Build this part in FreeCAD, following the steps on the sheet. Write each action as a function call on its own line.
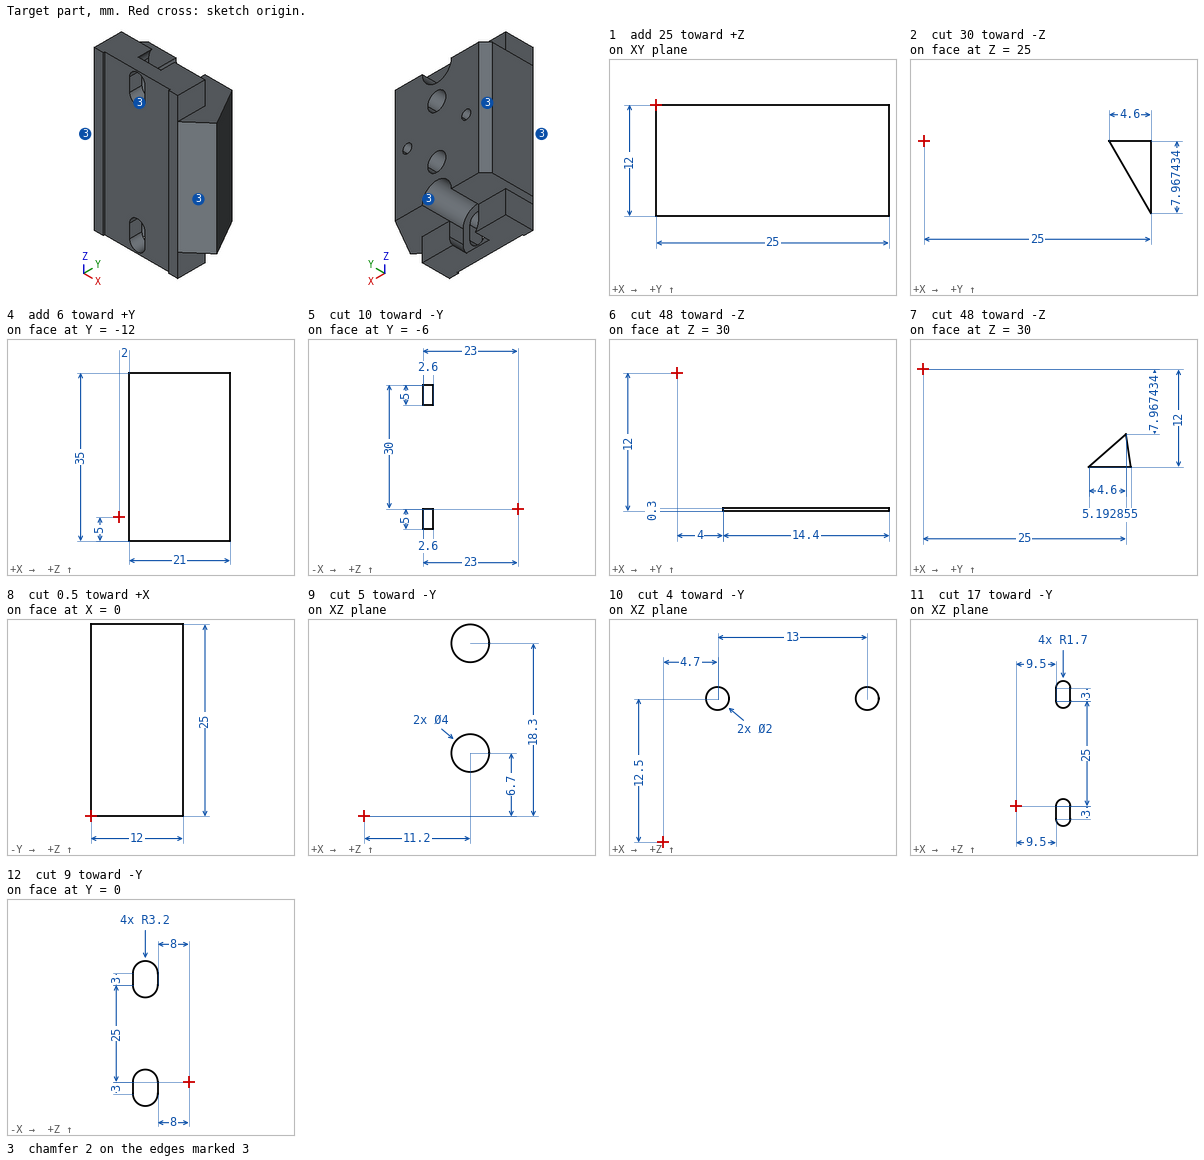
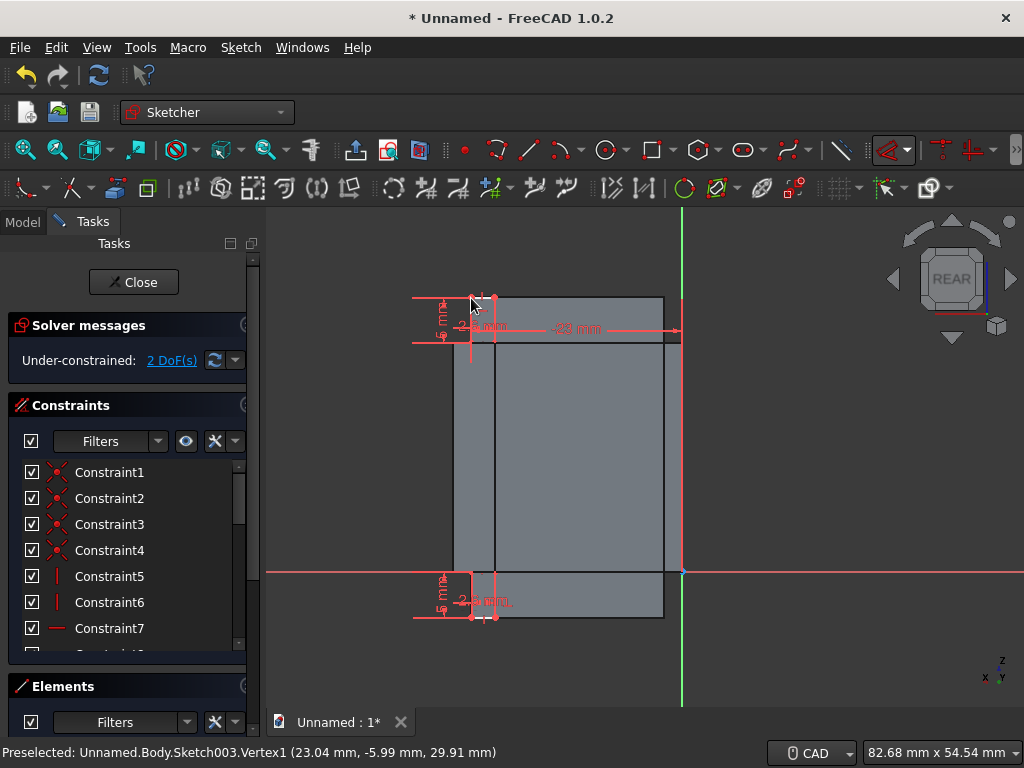
click(471, 298)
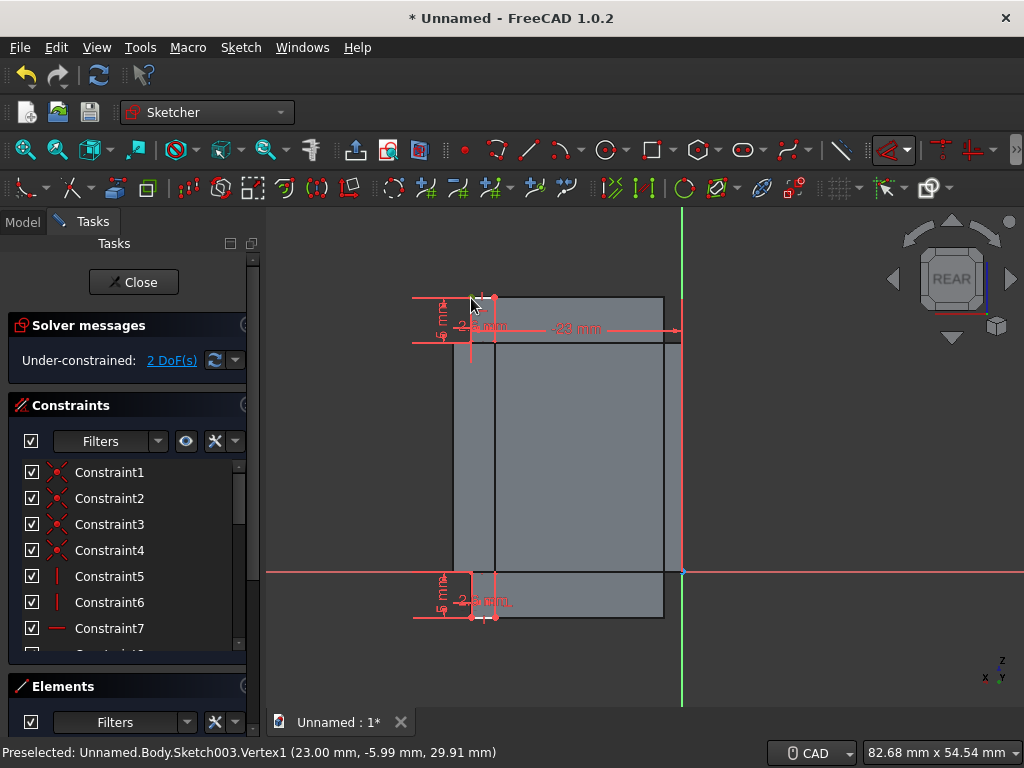
click(910, 150)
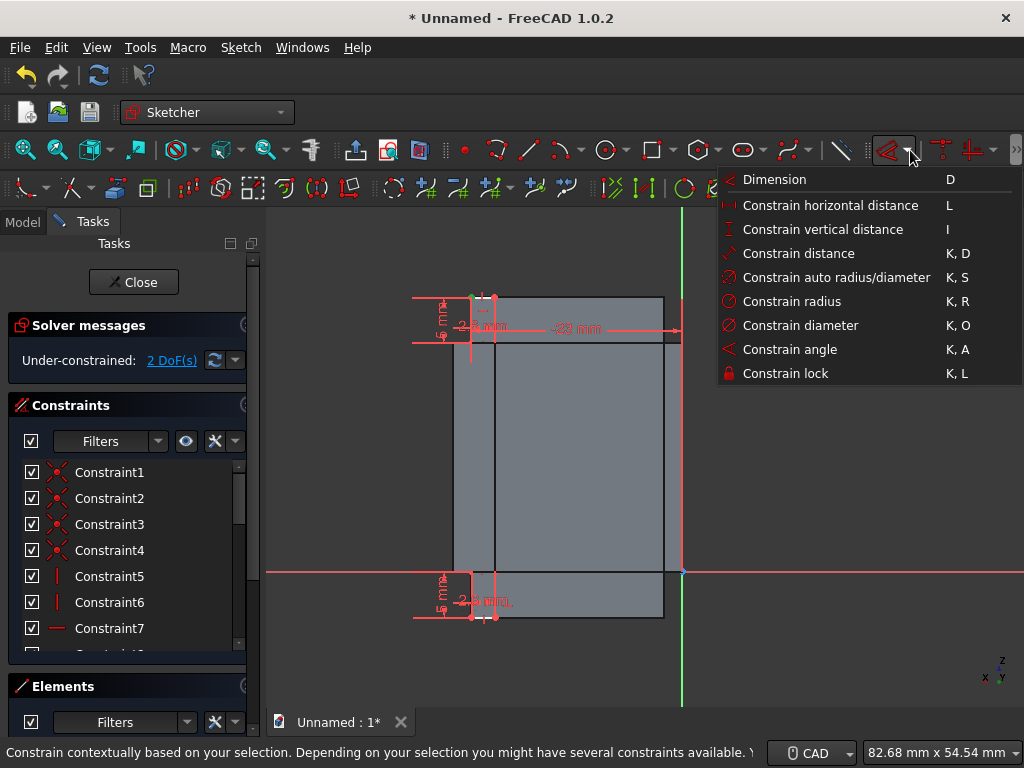
click(870, 229)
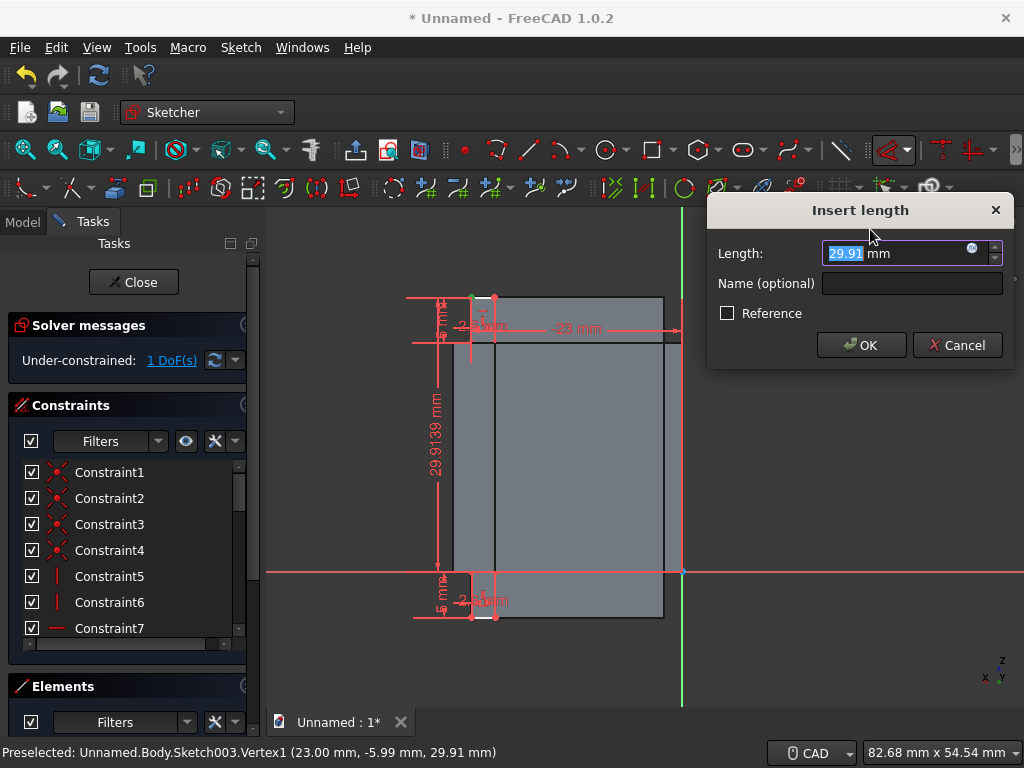
text(30)
key(Return)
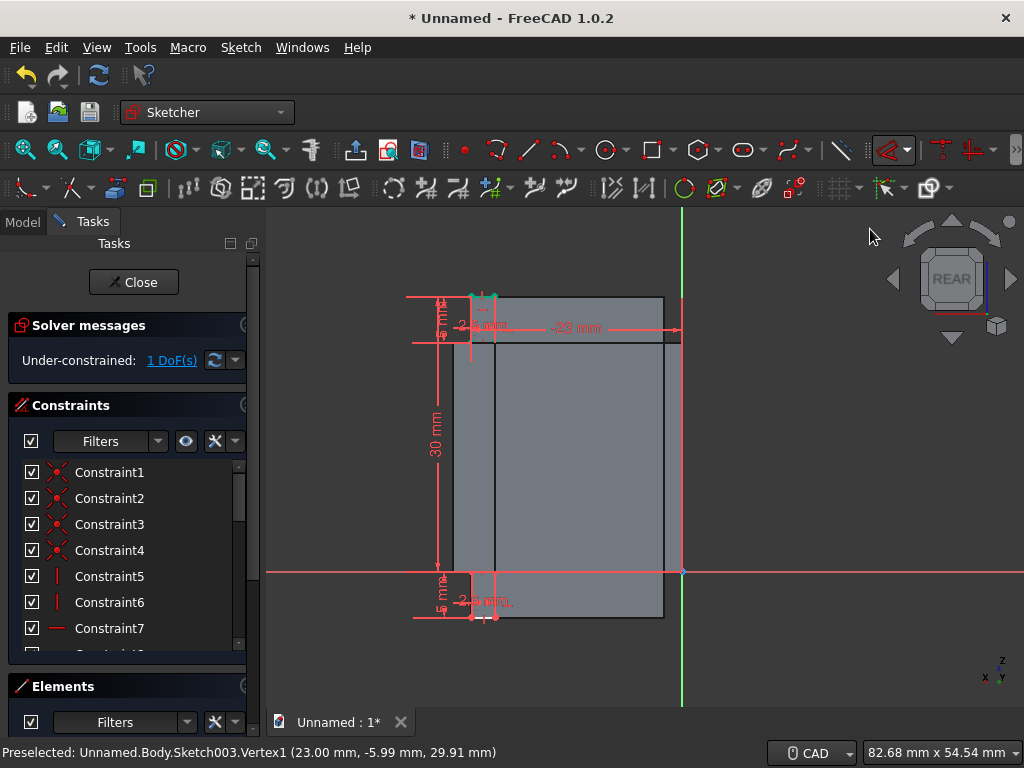
click(472, 572)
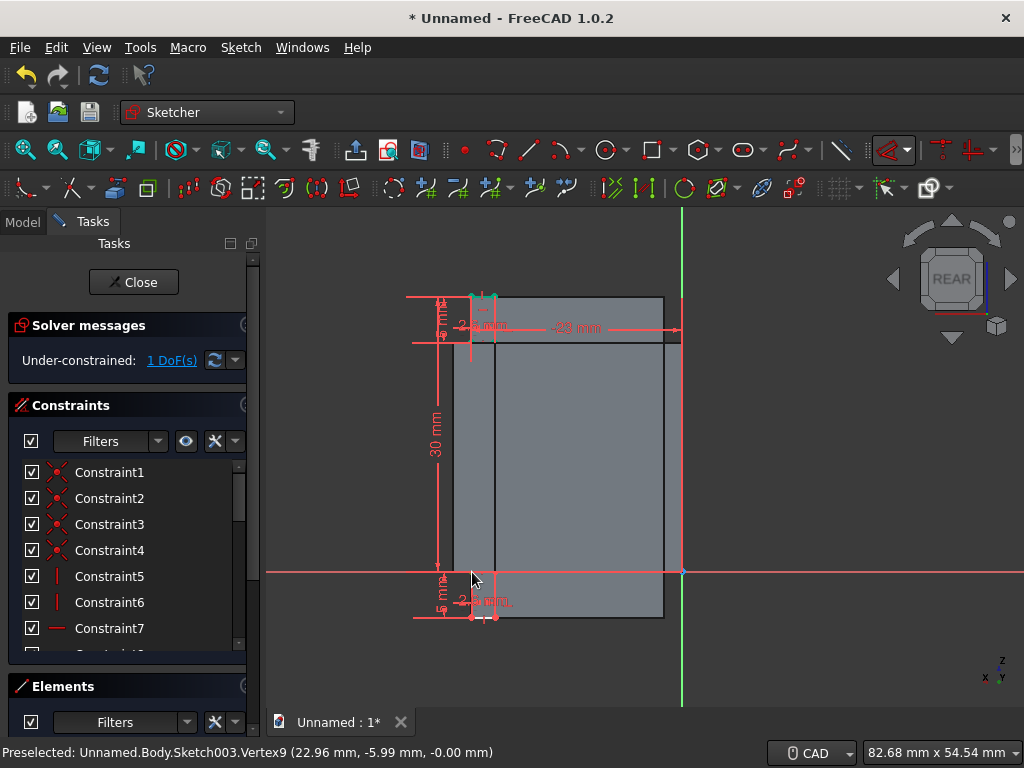
click(910, 150)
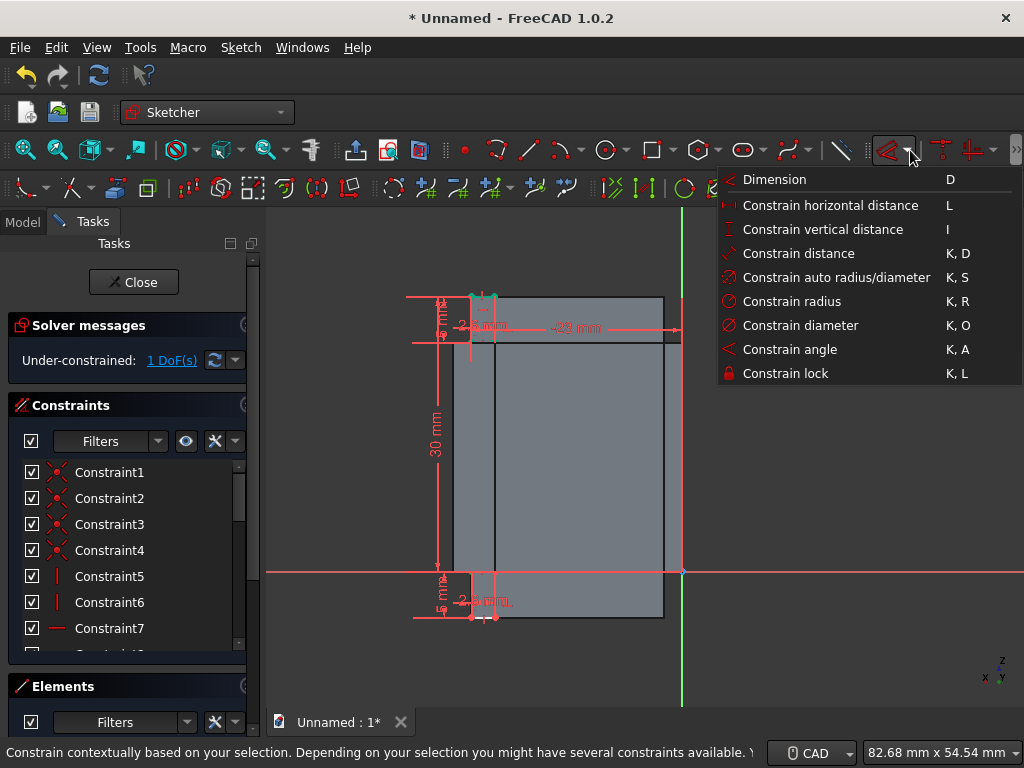
click(870, 205)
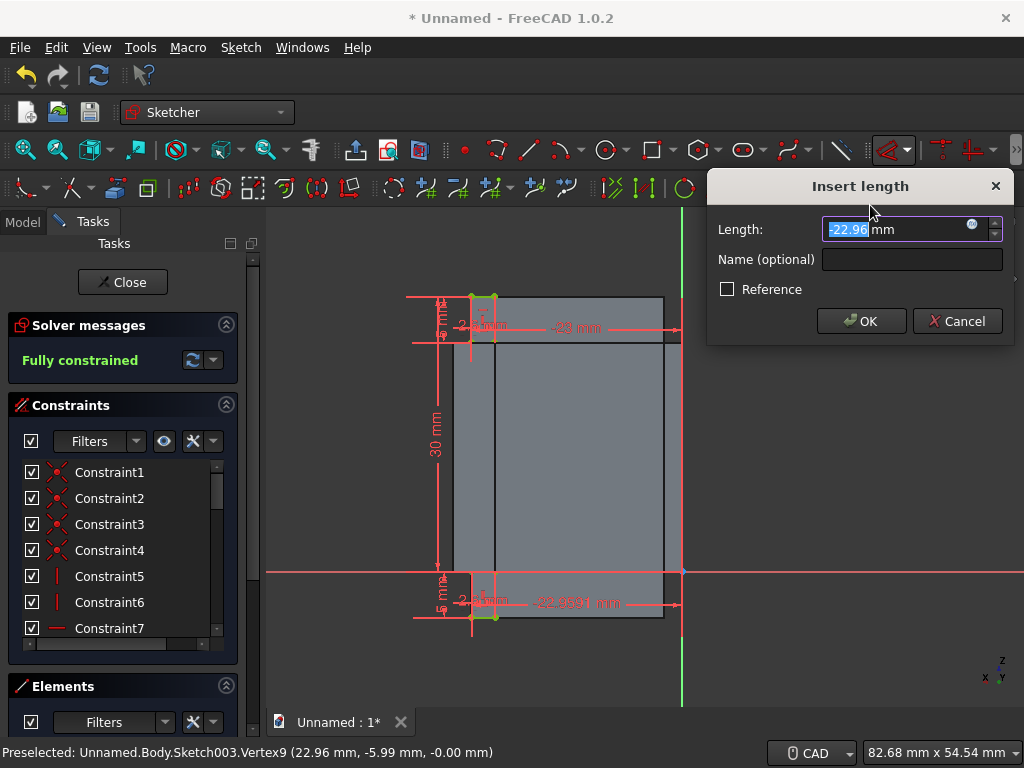
text(-23)
key(Return)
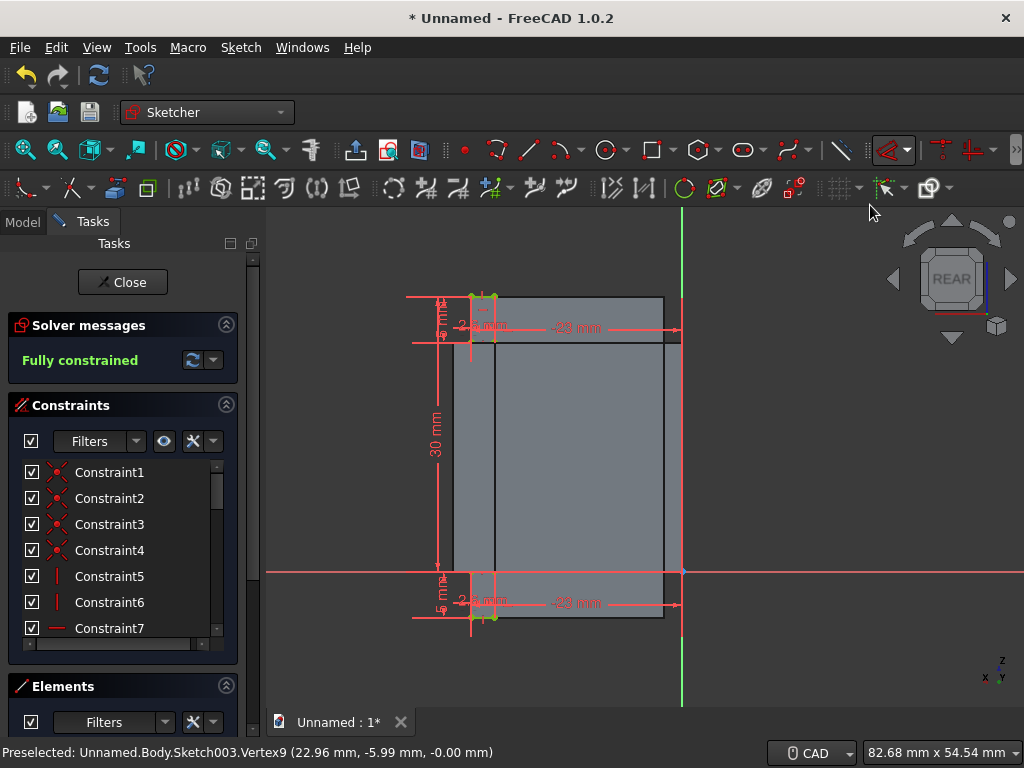
click(123, 282)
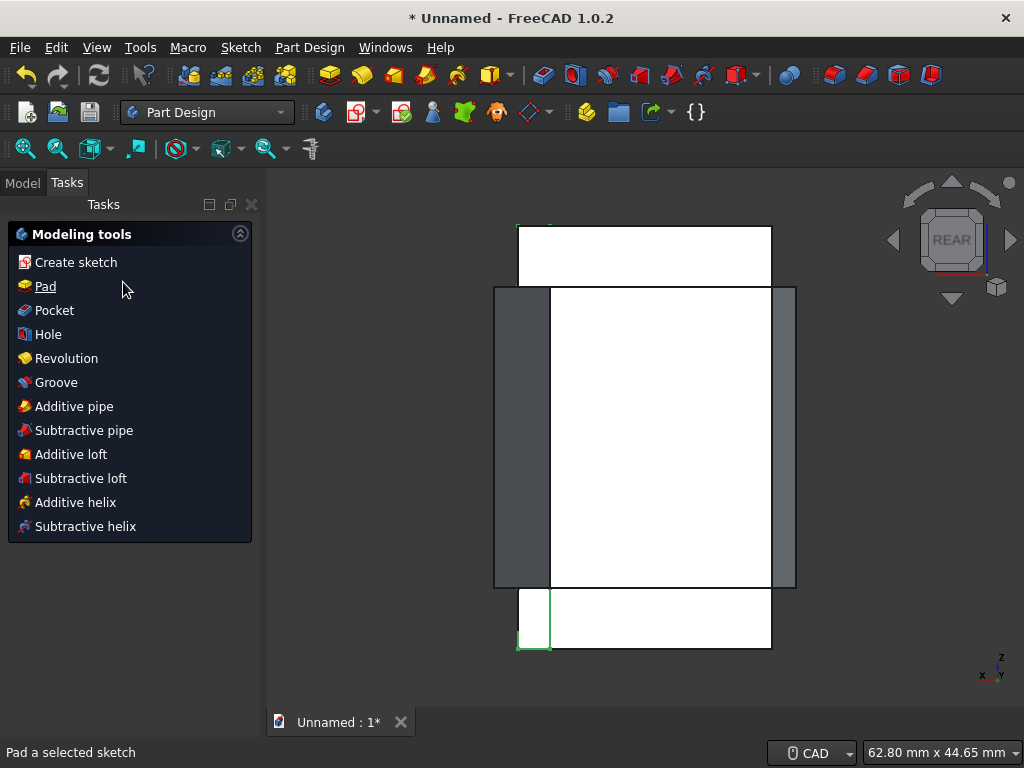
click(544, 76)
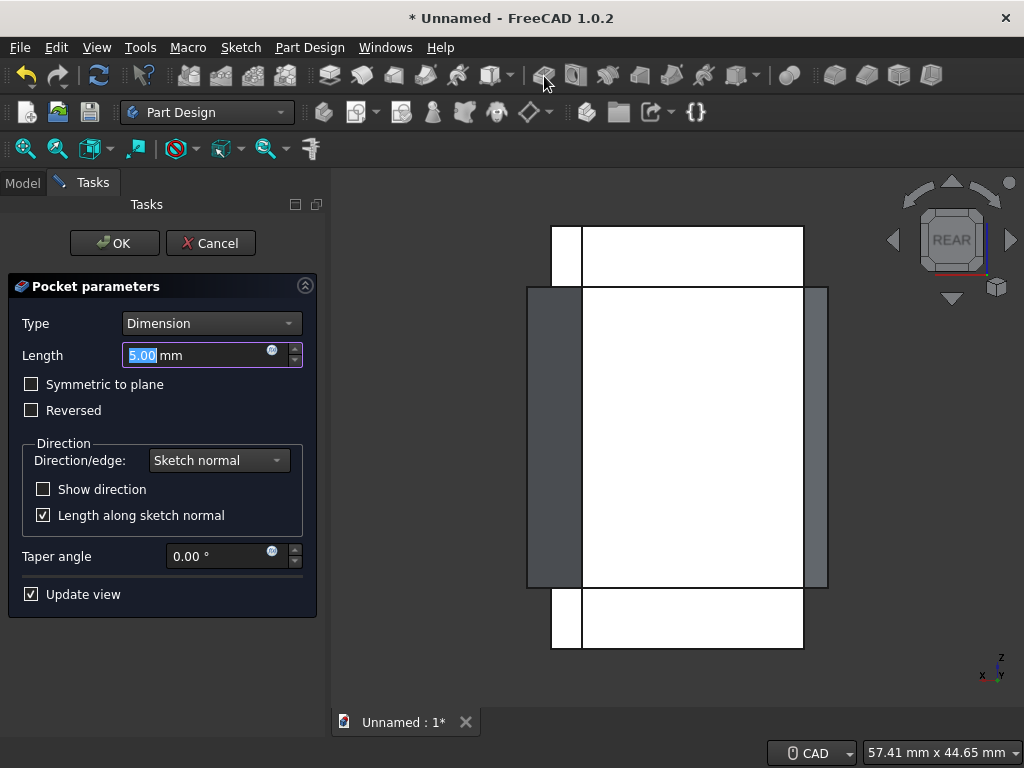
text(10)
key(Tab)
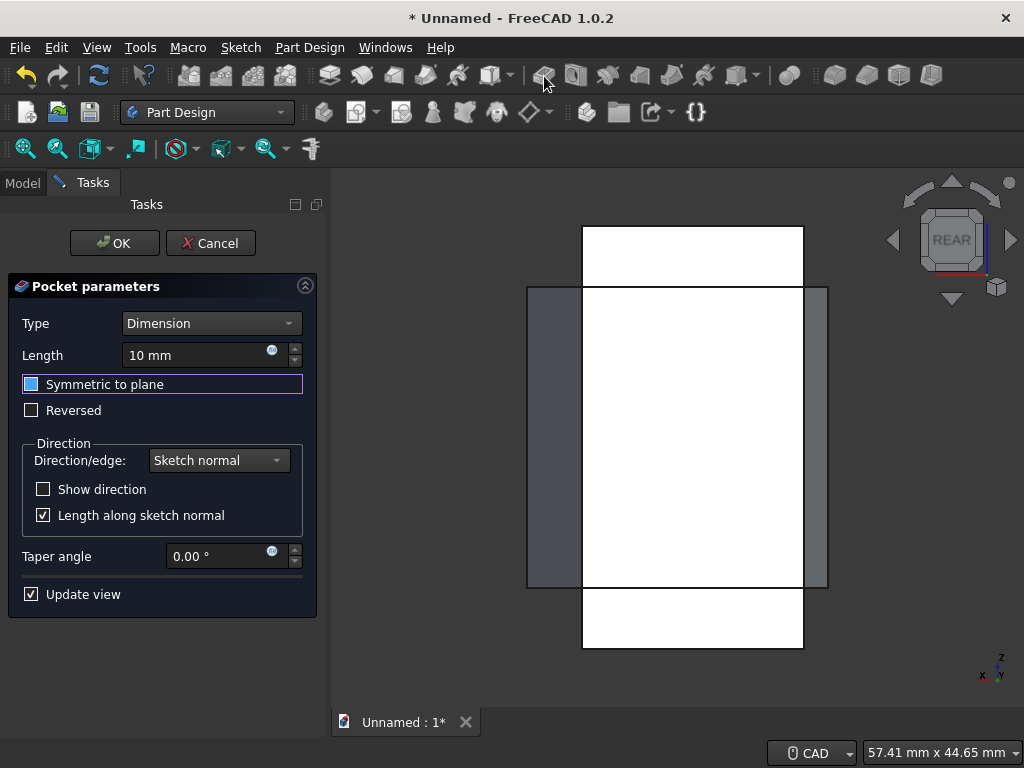
click(115, 243)